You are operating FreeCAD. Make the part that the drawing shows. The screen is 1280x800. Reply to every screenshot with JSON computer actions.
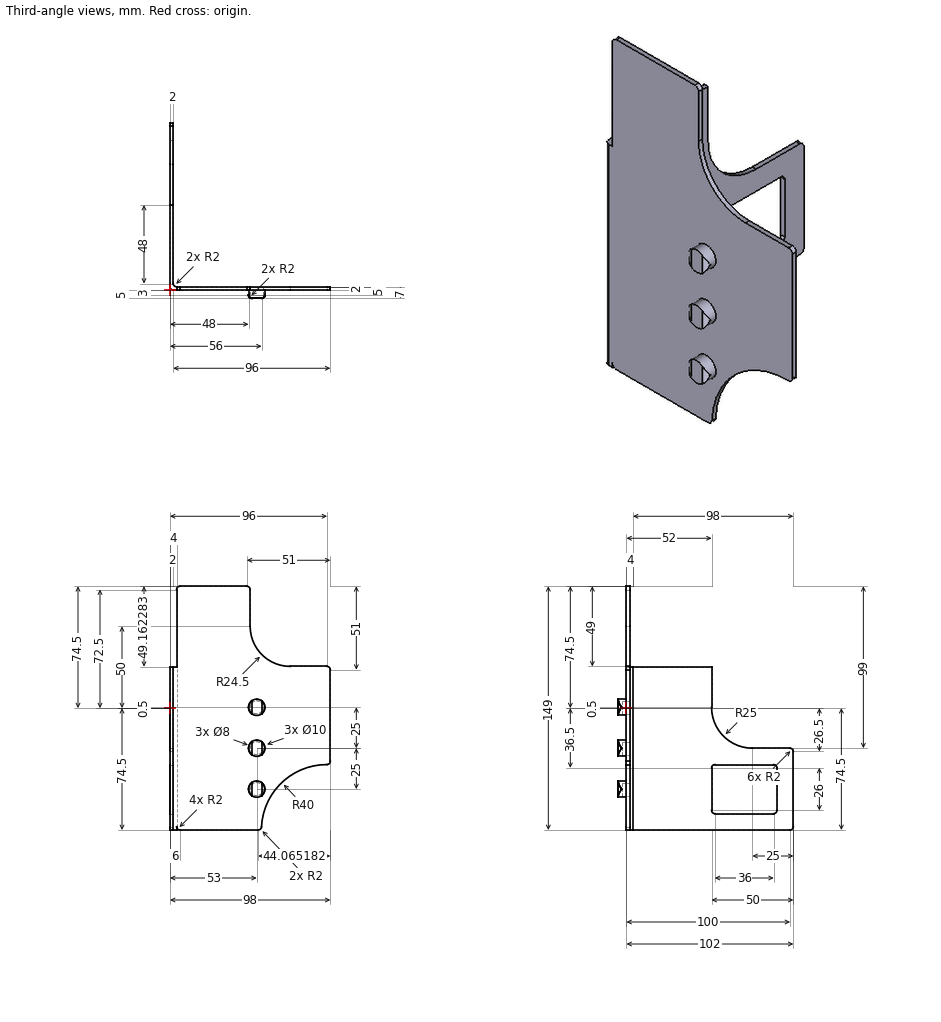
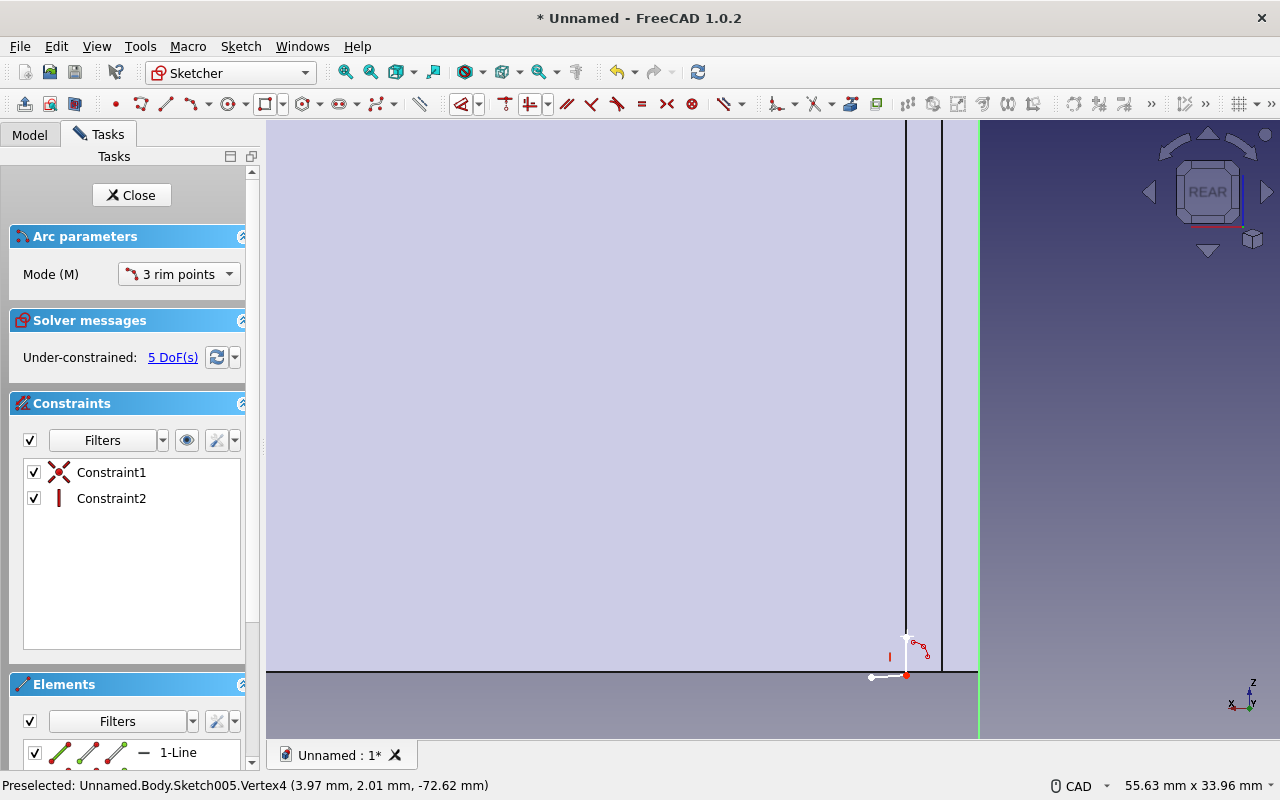
{"action": "left_click", "coordinate": [906, 637]}
{"action": "left_click", "coordinate": [872, 678]}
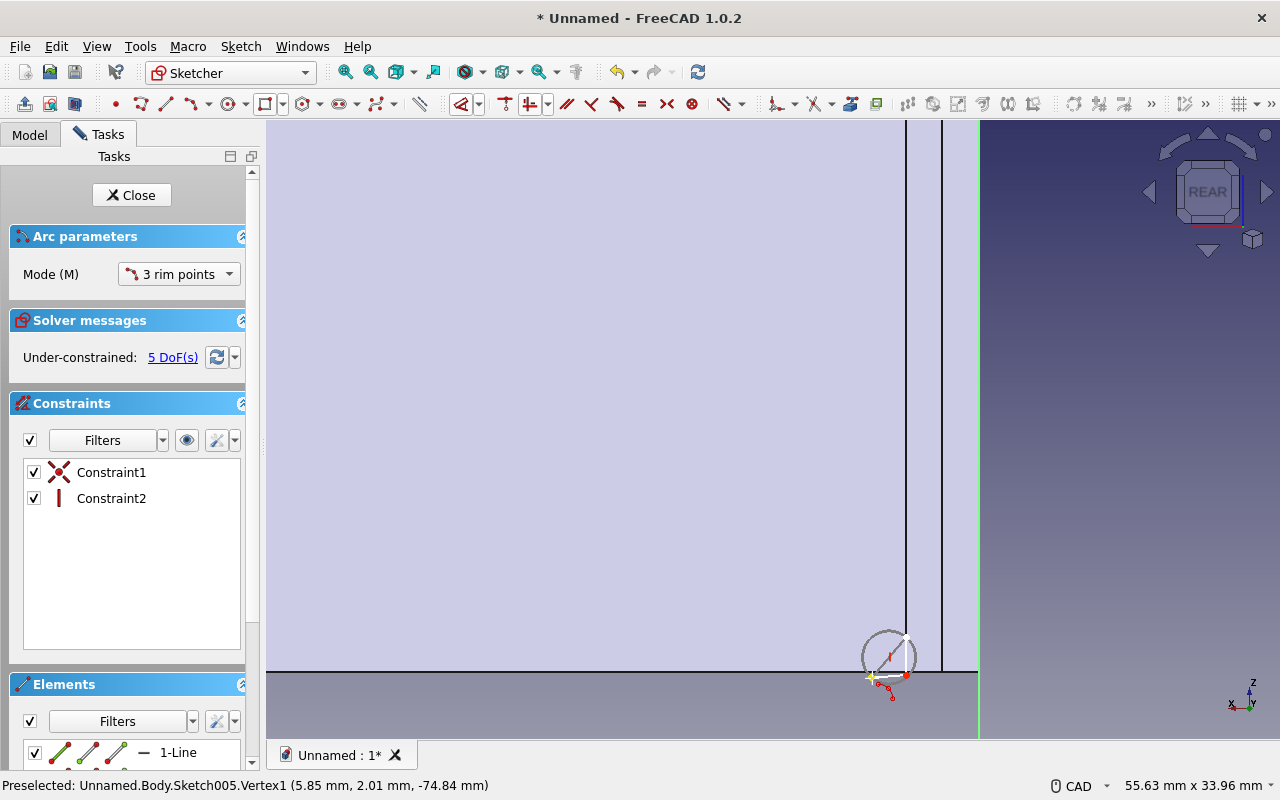
{"action": "scroll", "coordinate": [895, 661], "scroll_direction": "up", "scroll_amount": 2}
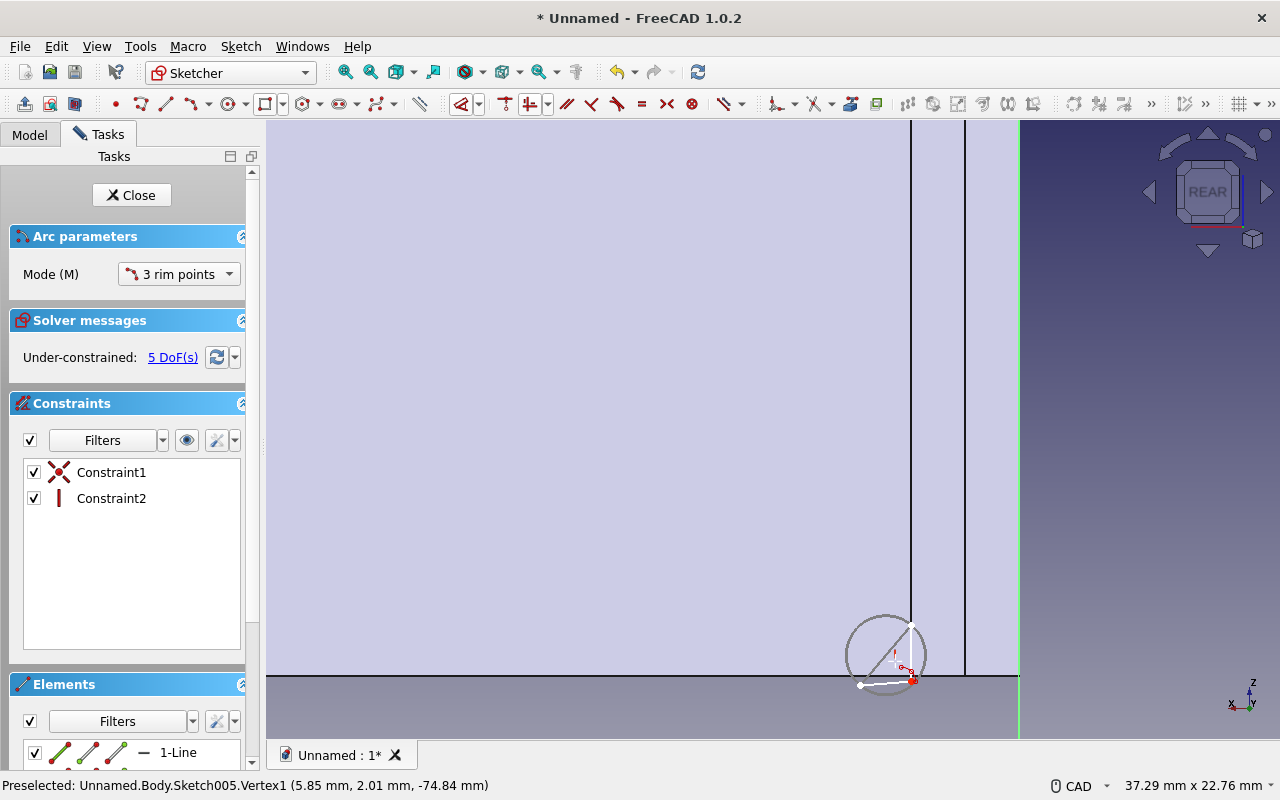
{"action": "left_click", "coordinate": [895, 660]}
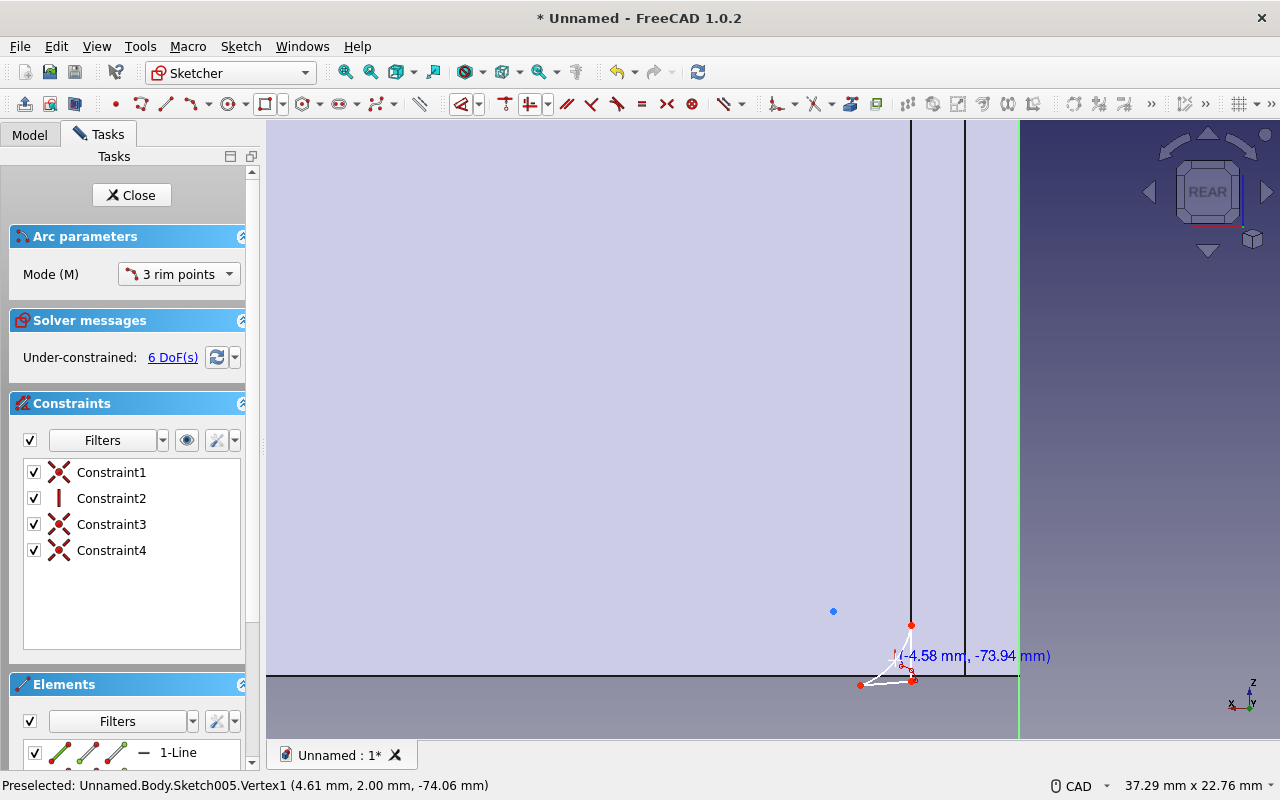
{"action": "key", "text": "g l"}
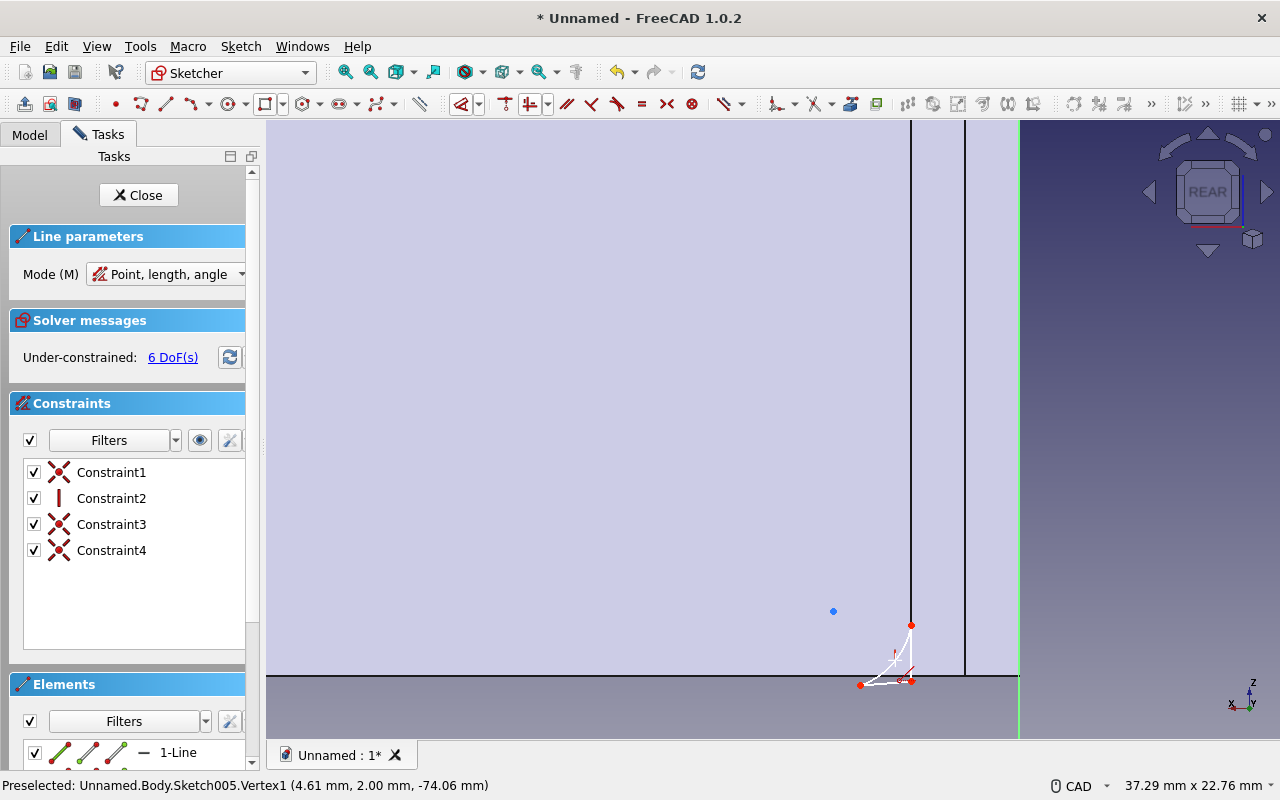
{"action": "scroll", "coordinate": [806, 607], "scroll_direction": "down", "scroll_amount": 12}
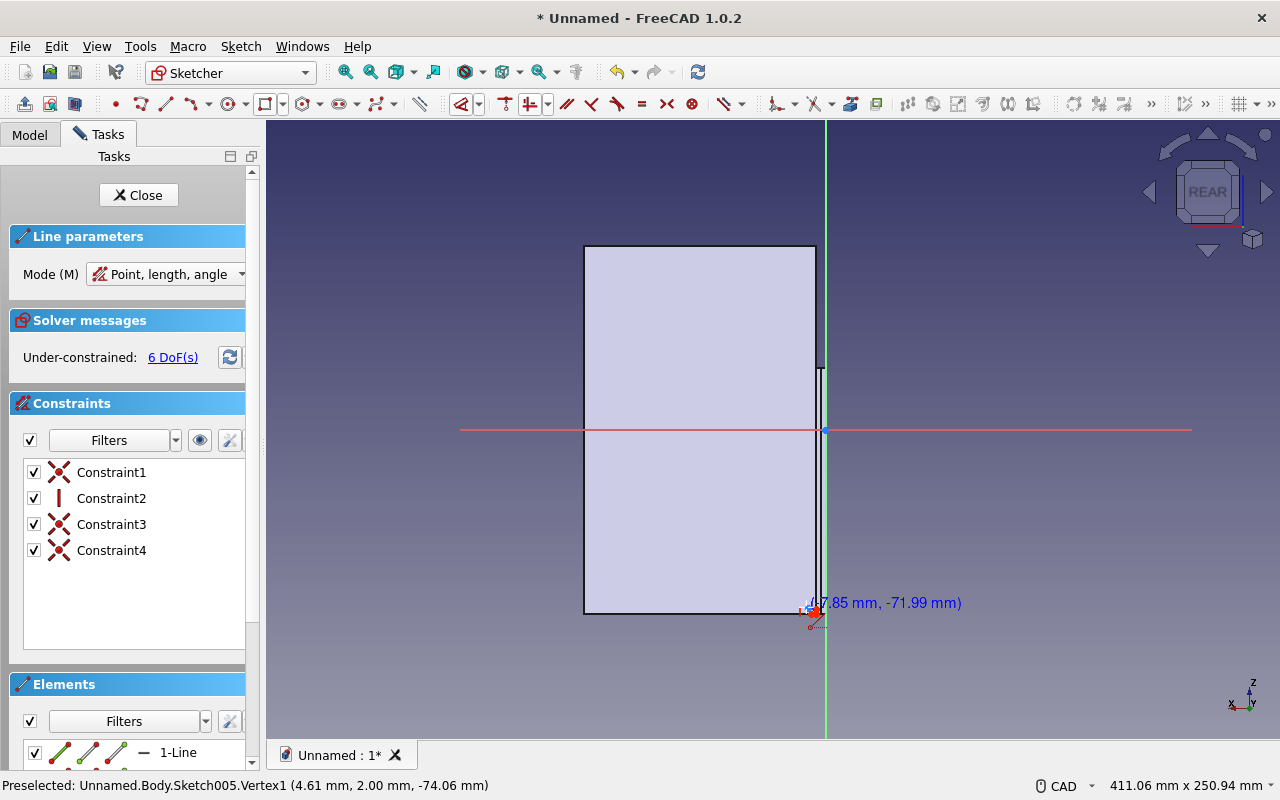
{"action": "left_click", "coordinate": [589, 367]}
{"action": "left_click", "coordinate": [645, 367]}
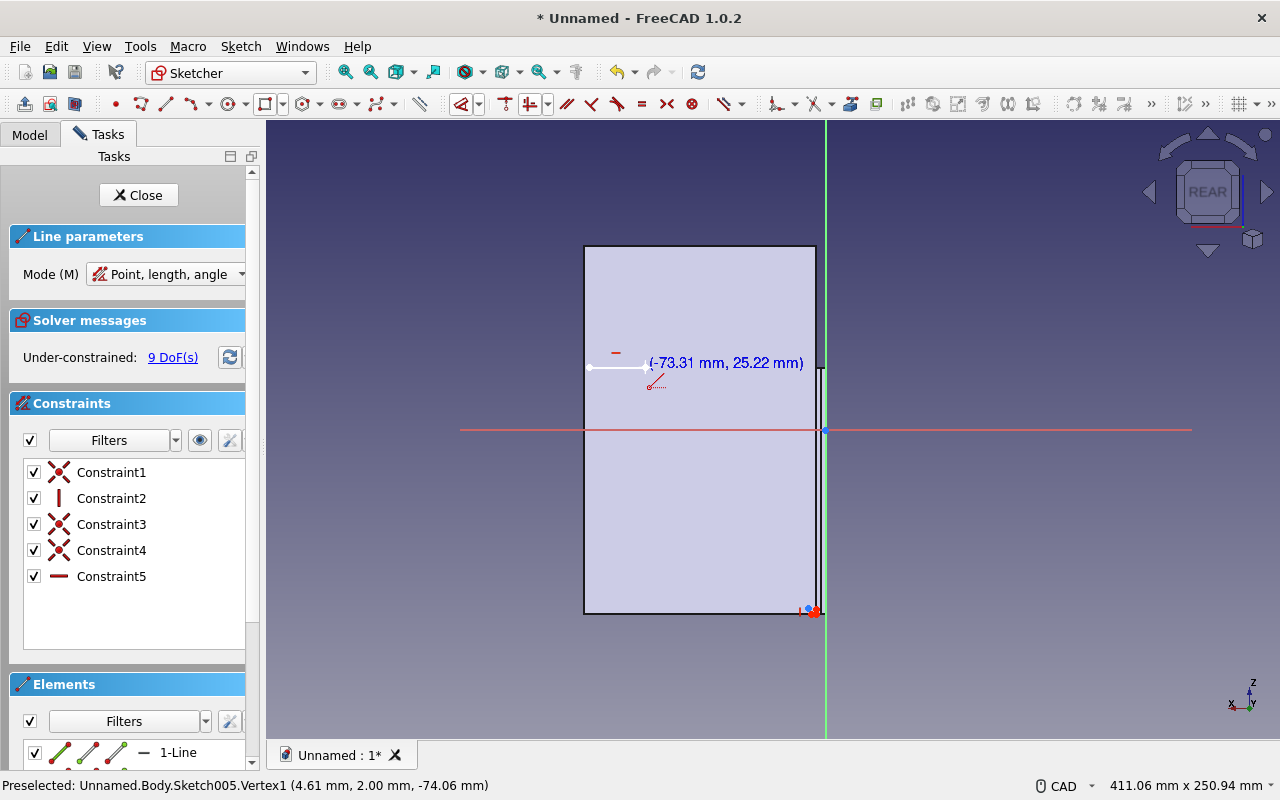
{"action": "left_click", "coordinate": [705, 307]}
{"action": "left_click", "coordinate": [705, 251]}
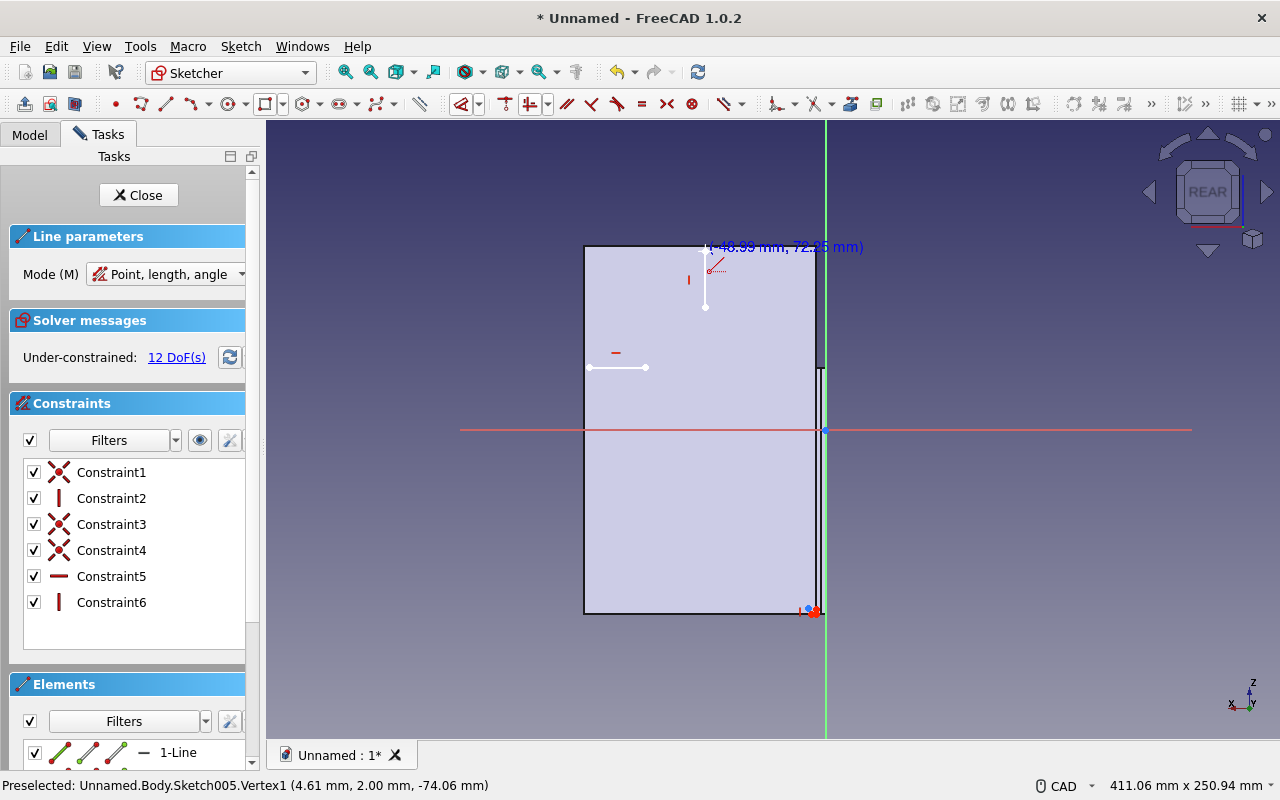
{"action": "left_click", "coordinate": [141, 104]}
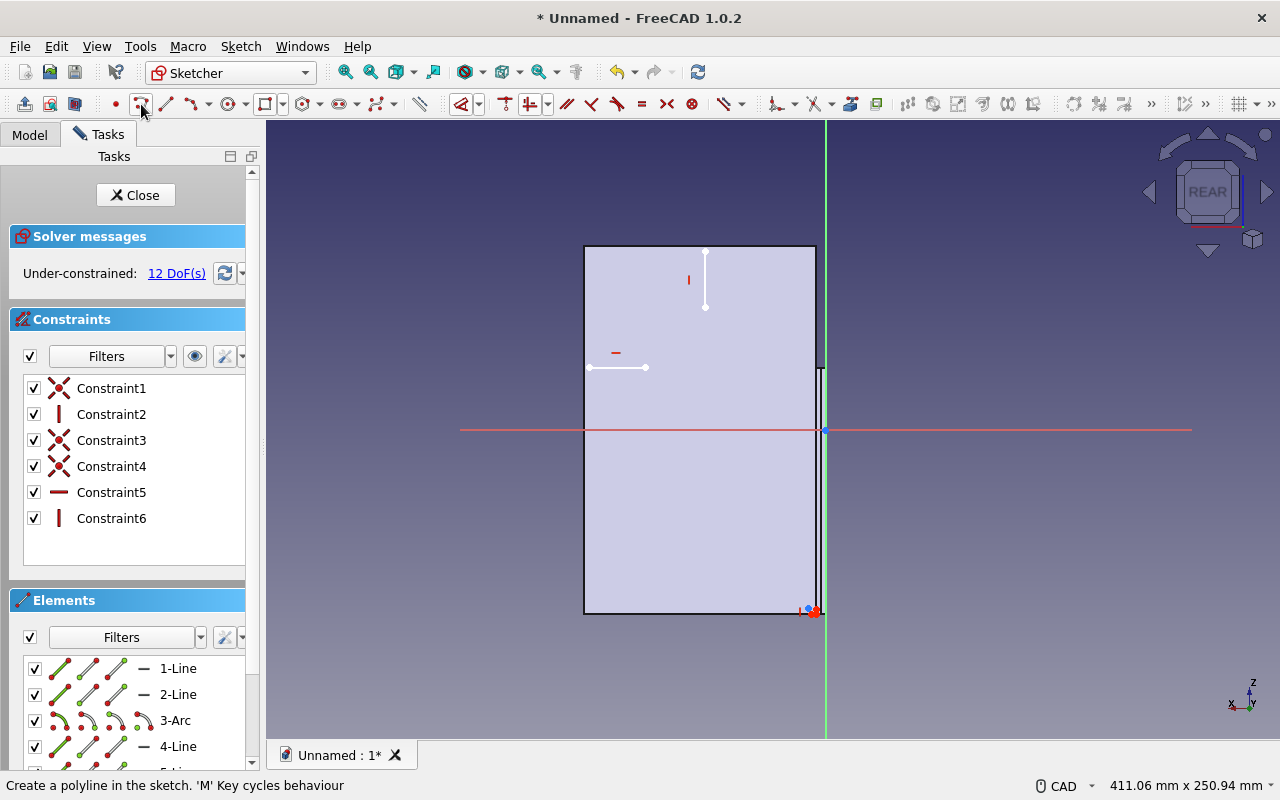
{"action": "scroll", "coordinate": [710, 246], "scroll_direction": "up", "scroll_amount": 5}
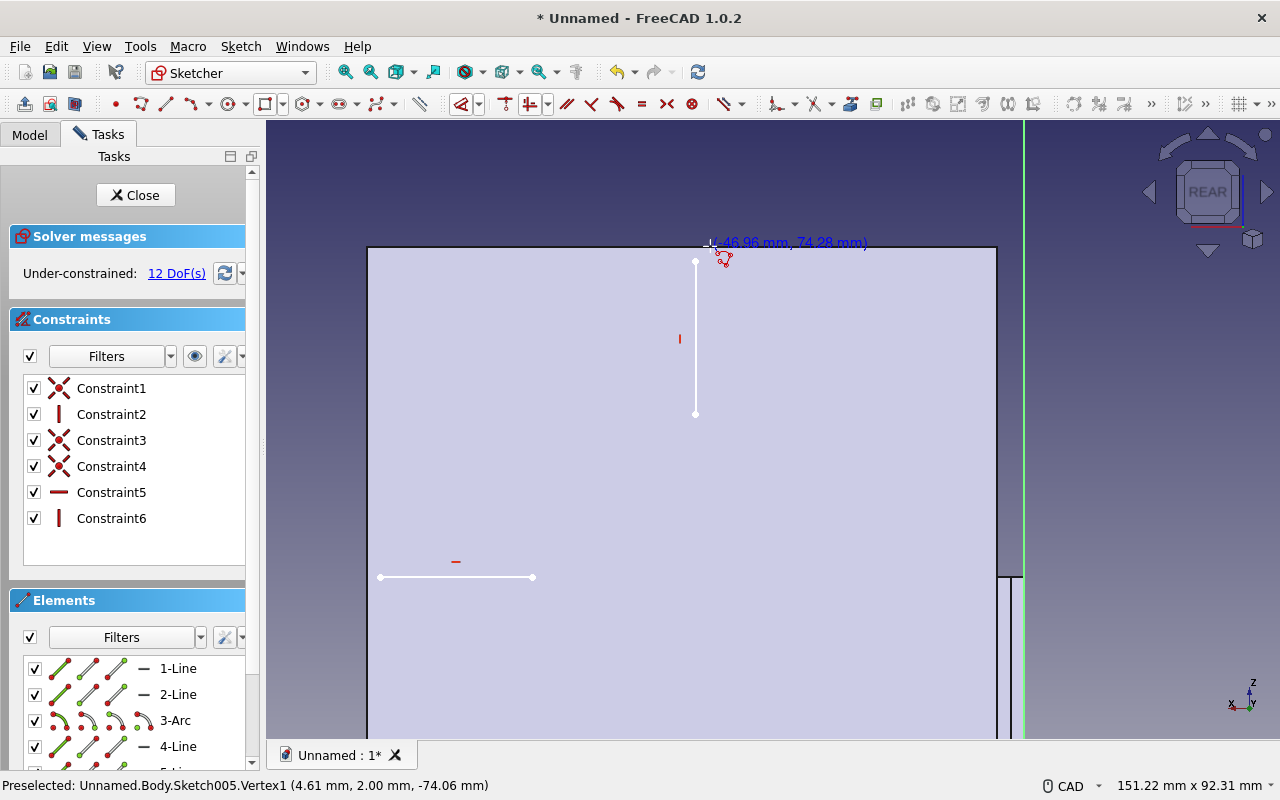
{"action": "left_click", "coordinate": [709, 247]}
{"action": "left_click", "coordinate": [367, 247]}
{"action": "left_click", "coordinate": [367, 589]}
{"action": "right_click", "coordinate": [367, 589]}